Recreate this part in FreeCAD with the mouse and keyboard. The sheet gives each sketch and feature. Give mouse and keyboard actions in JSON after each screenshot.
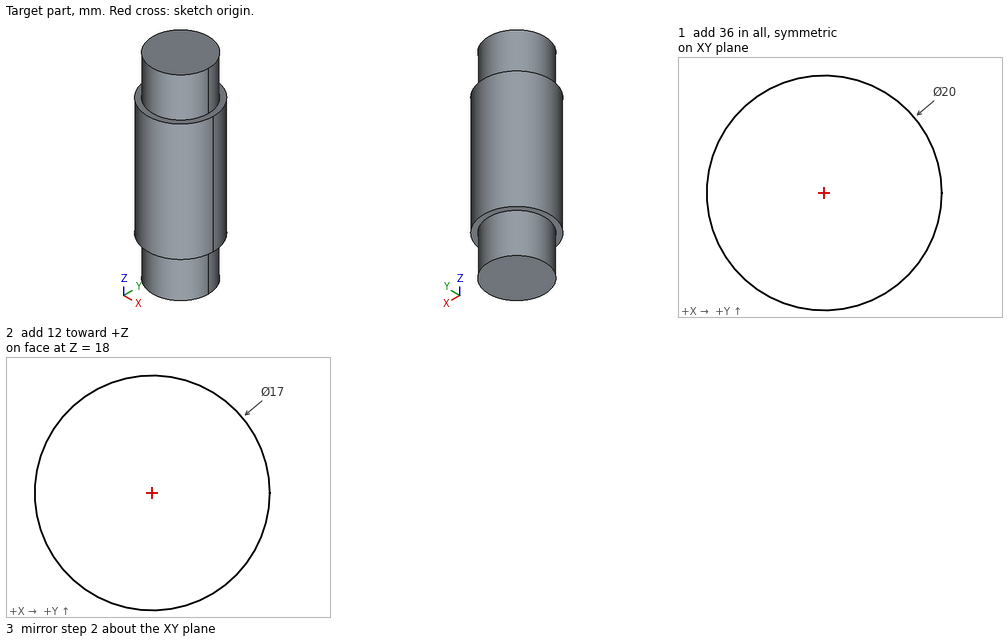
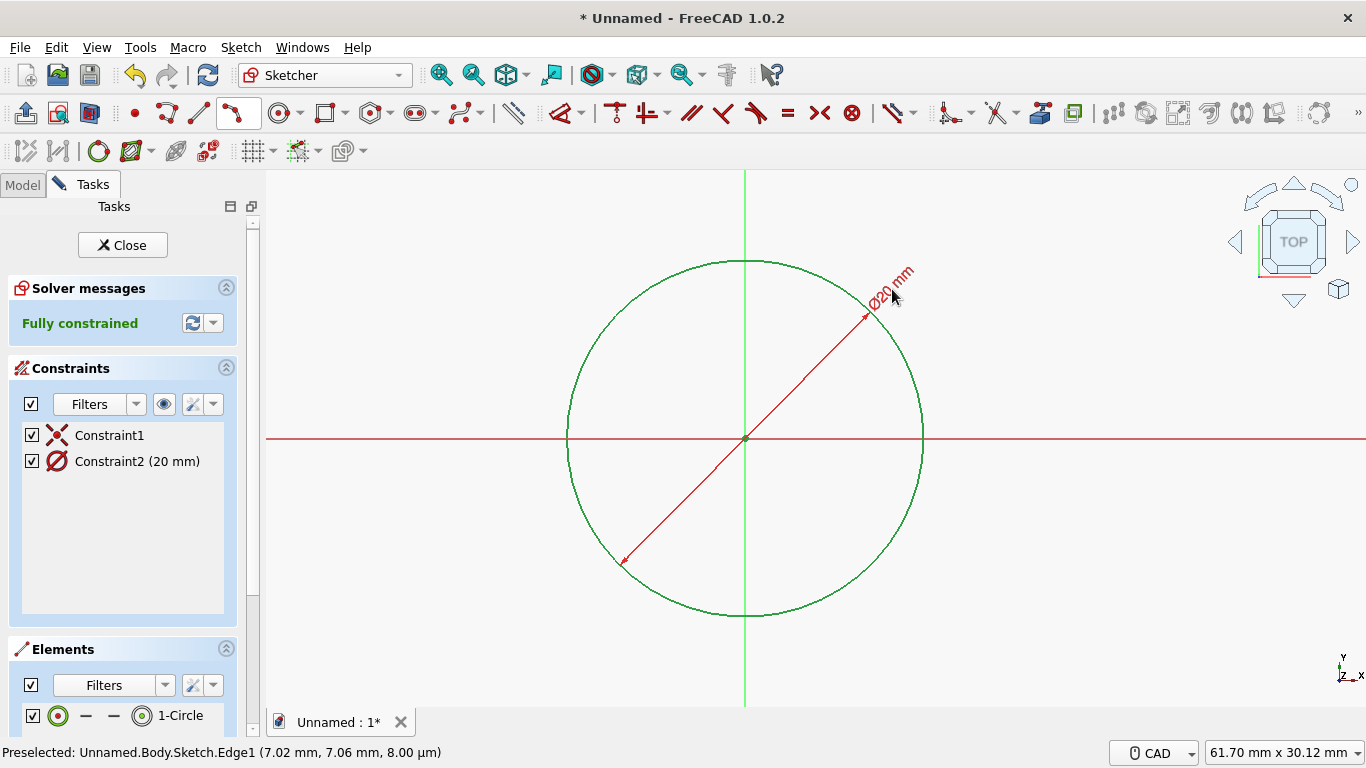
{"action": "left_click", "coordinate": [123, 245]}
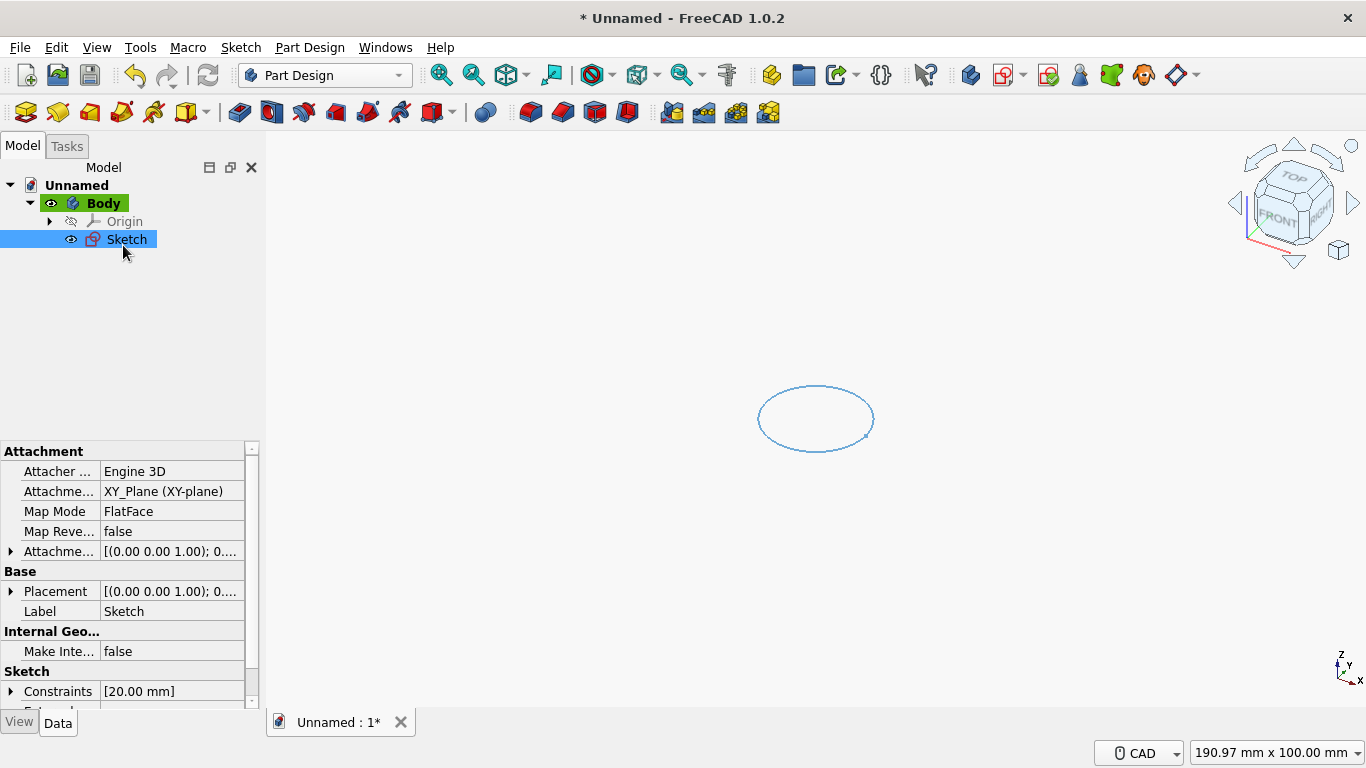
{"action": "left_click", "coordinate": [26, 112]}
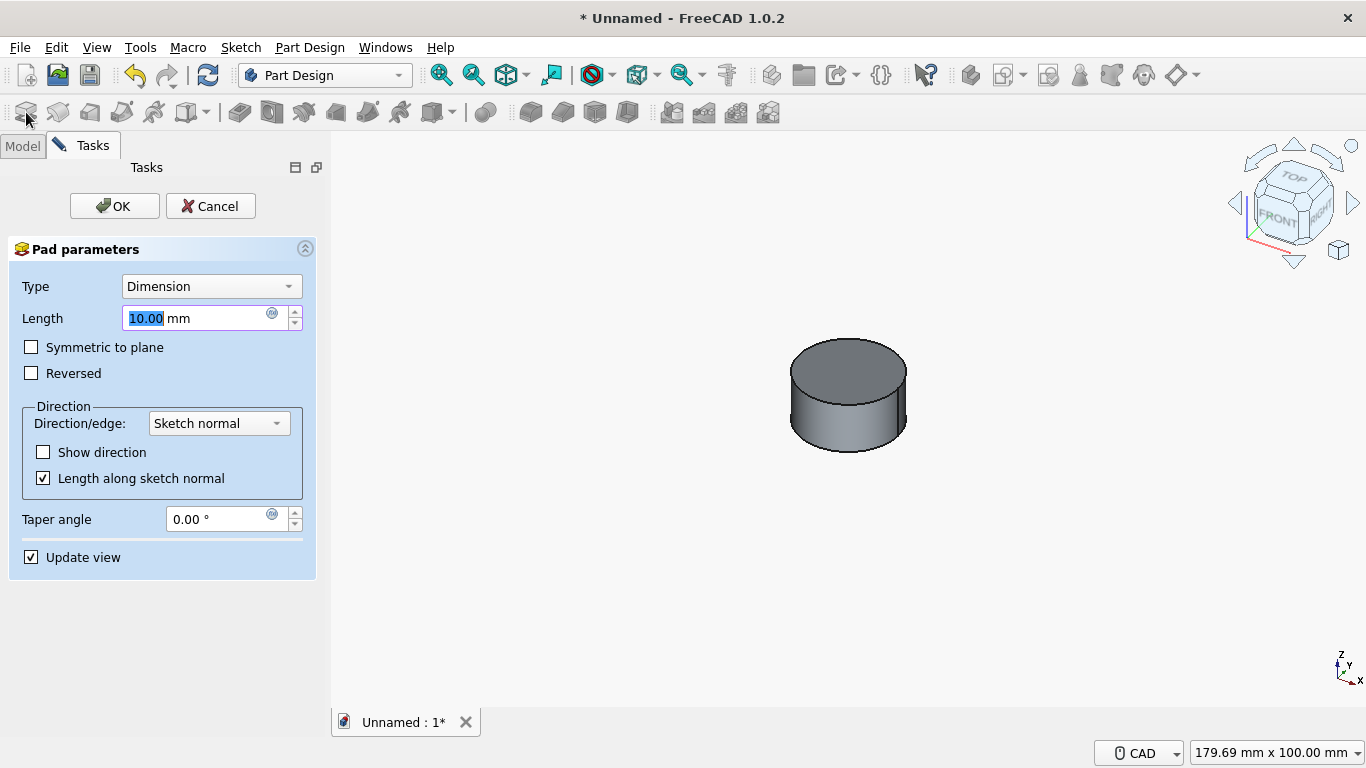
{"action": "type", "text": "36"}
{"action": "key", "text": "Tab"}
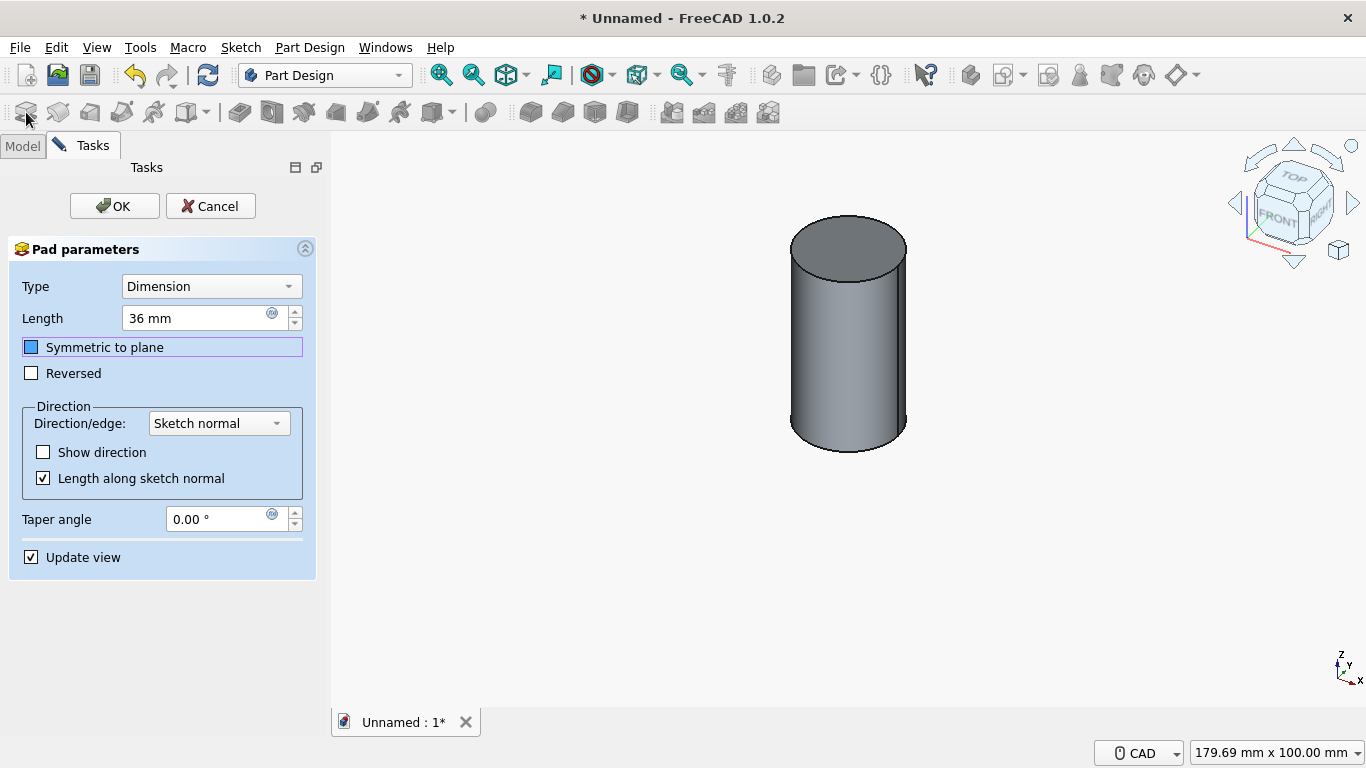
{"action": "left_click", "coordinate": [30, 347]}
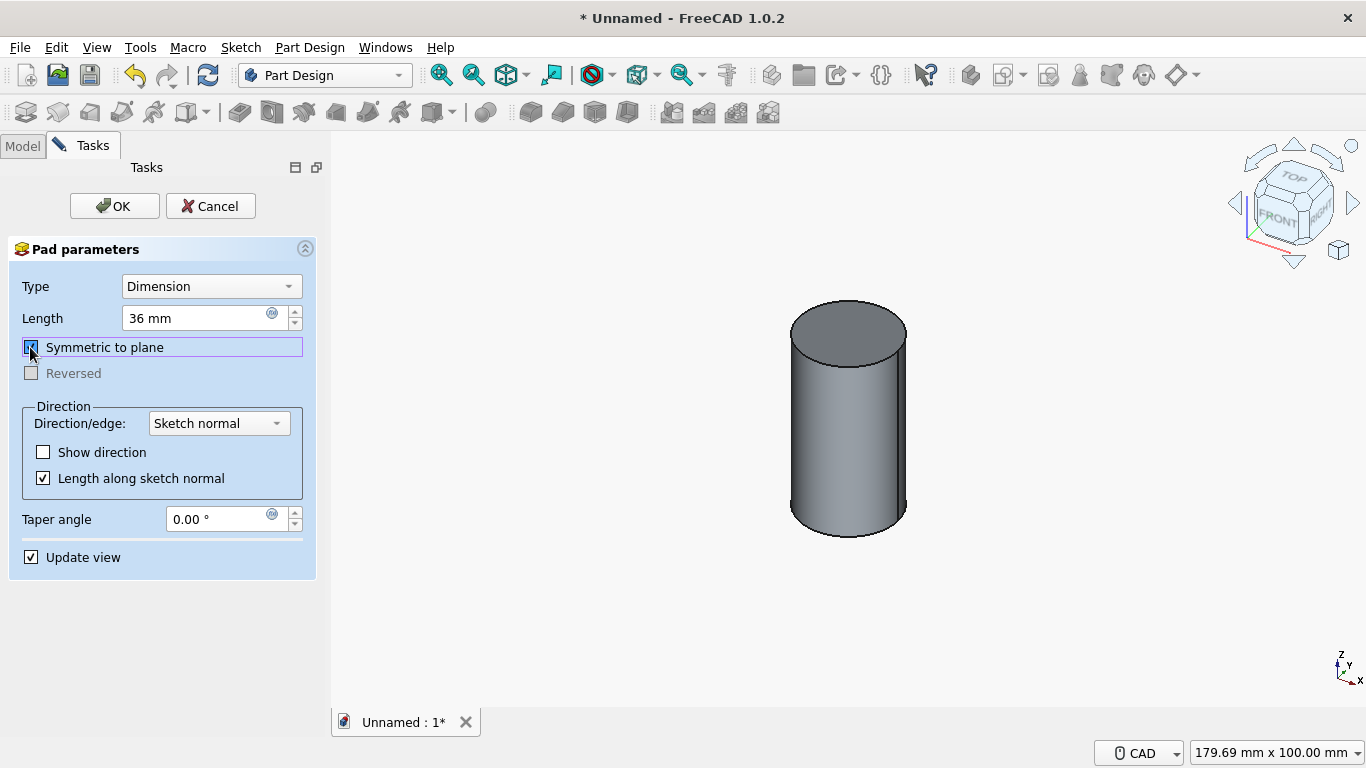
{"action": "left_click", "coordinate": [115, 206]}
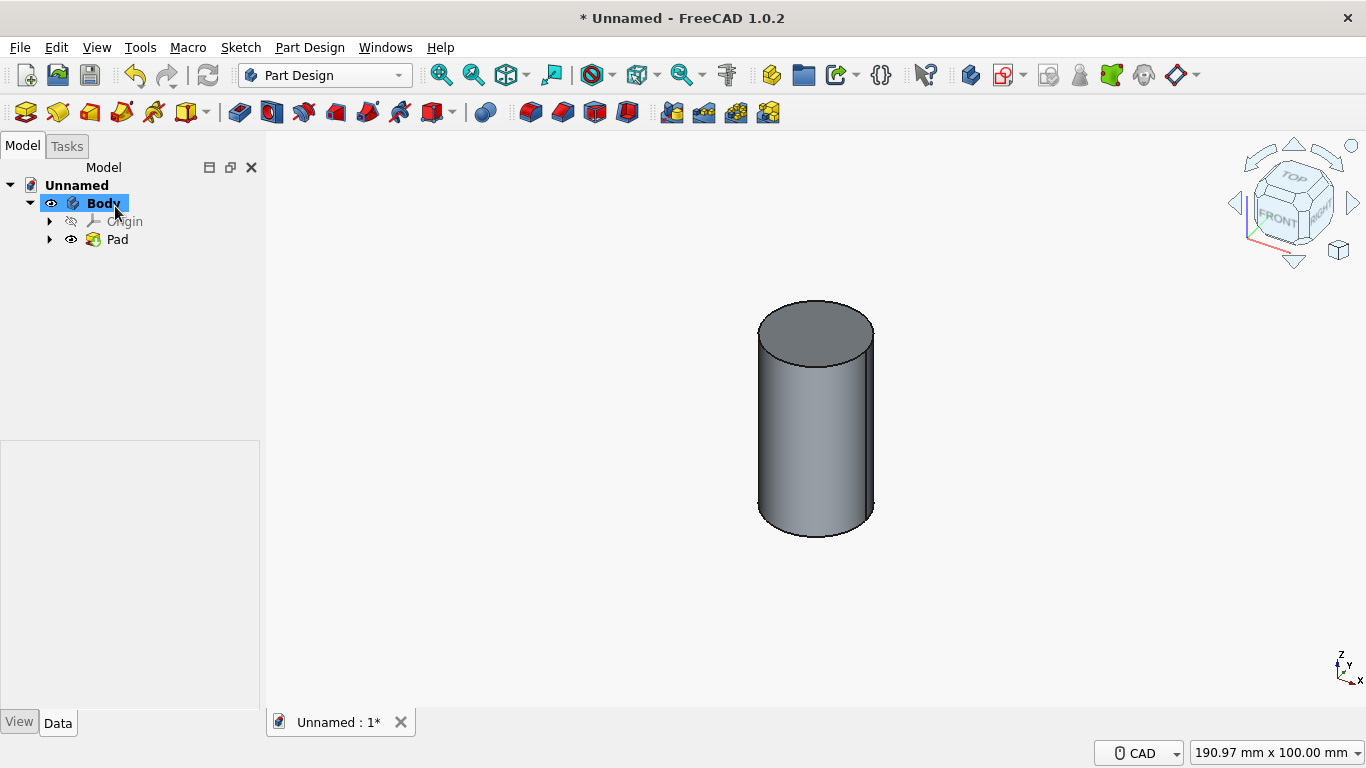
{"action": "left_click", "coordinate": [816, 333]}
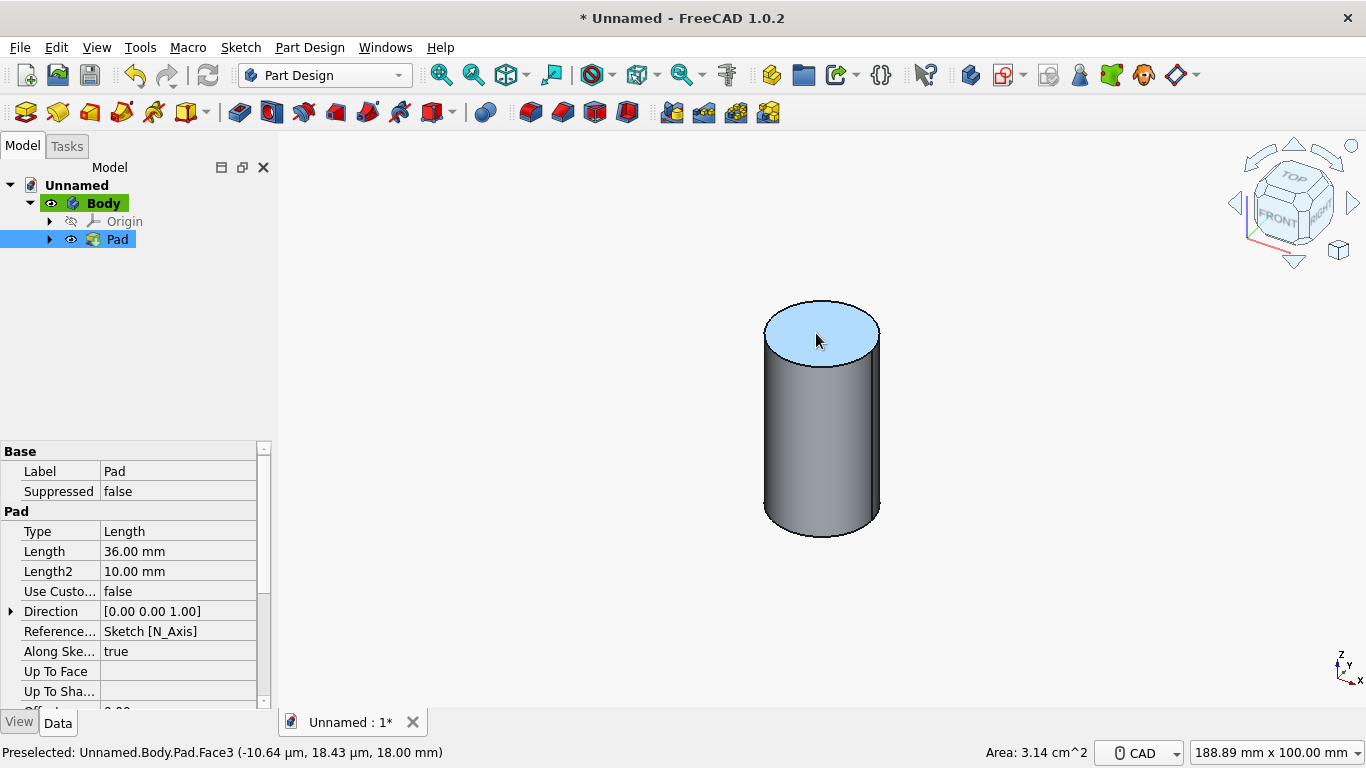
{"action": "left_click", "coordinate": [1004, 76]}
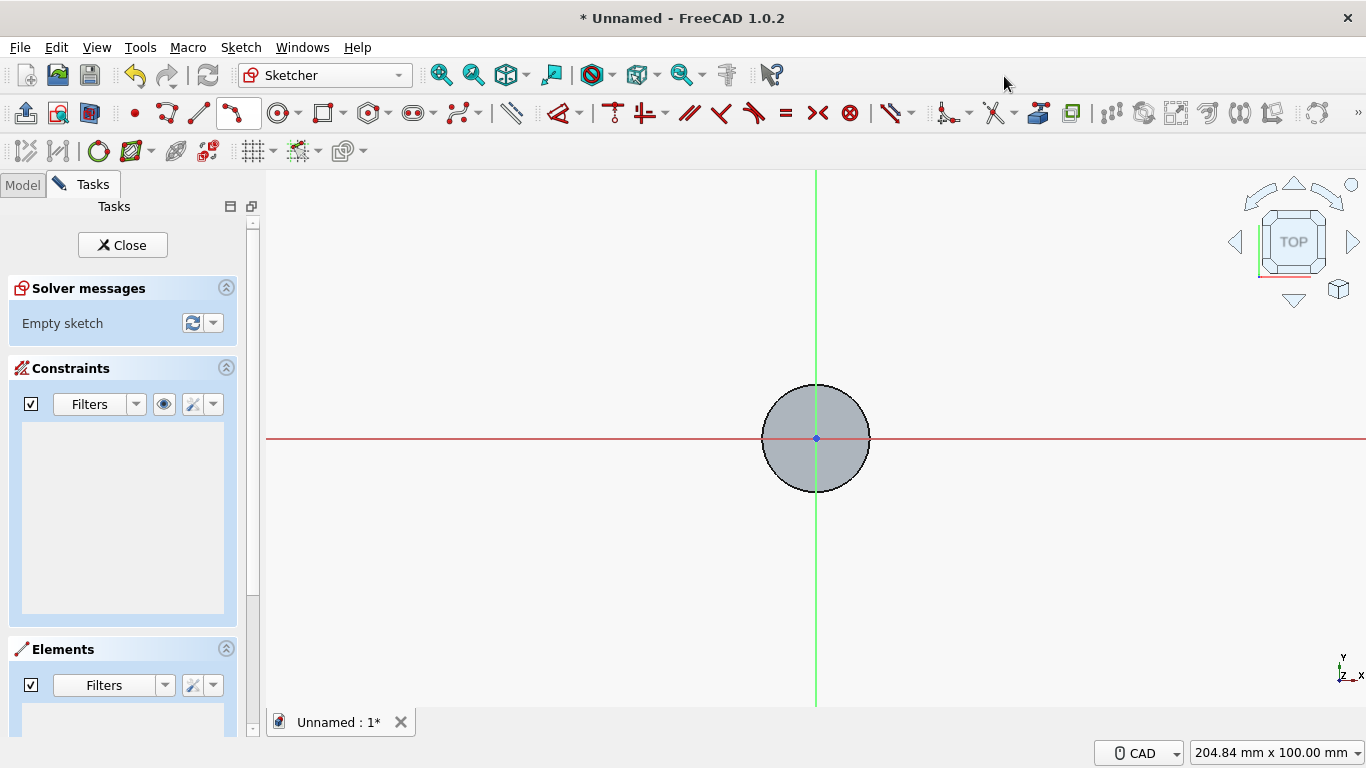
{"action": "scroll", "coordinate": [838, 438], "scroll_direction": "up", "scroll_amount": 7}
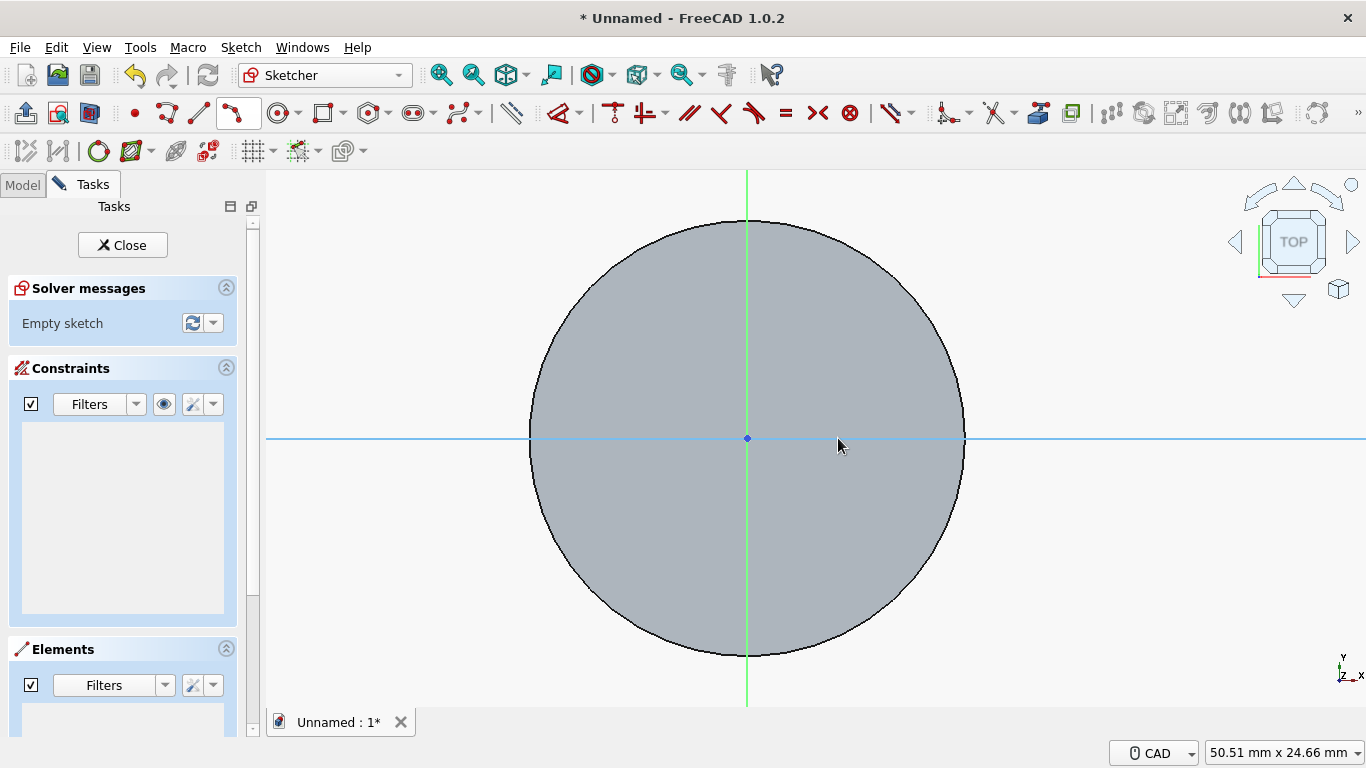
{"action": "left_click", "coordinate": [278, 114]}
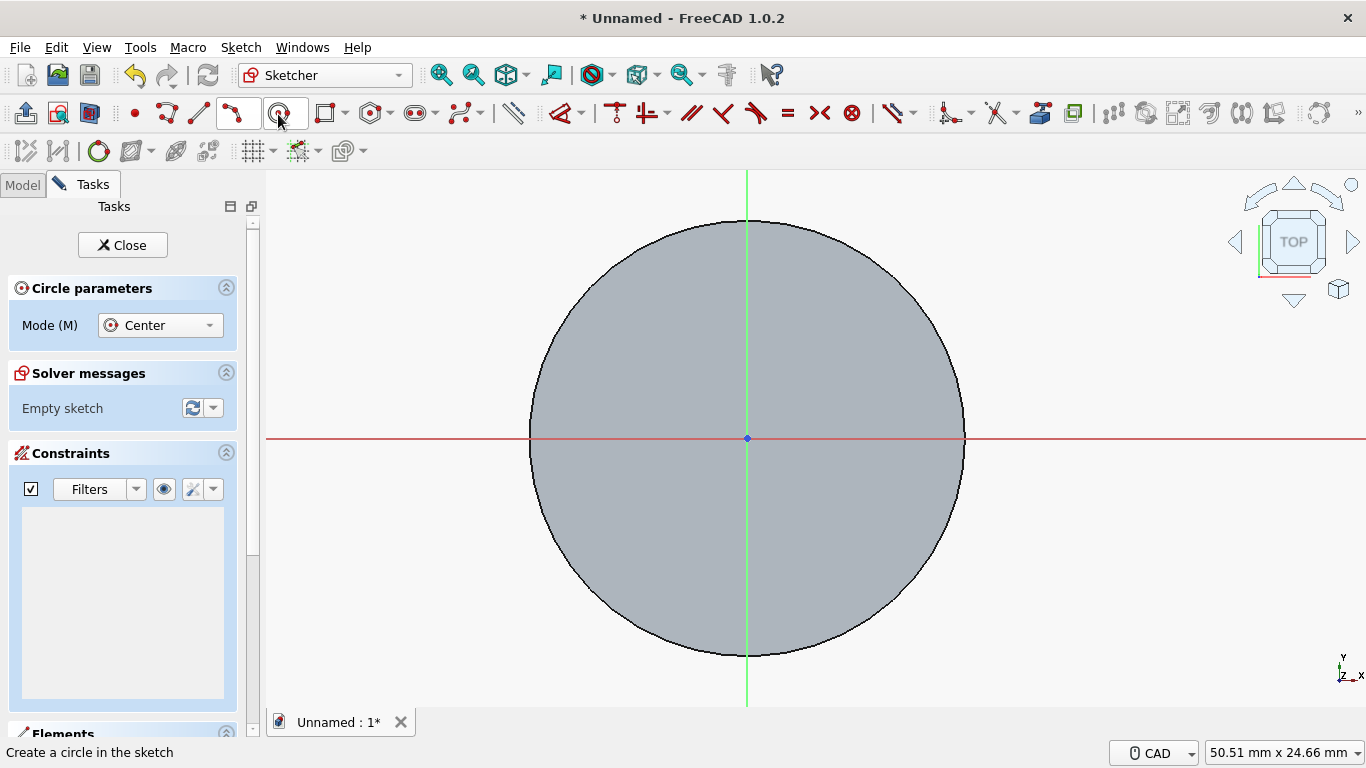
{"action": "left_click", "coordinate": [747, 438]}
{"action": "left_click", "coordinate": [878, 308]}
{"action": "key", "text": "Escape"}